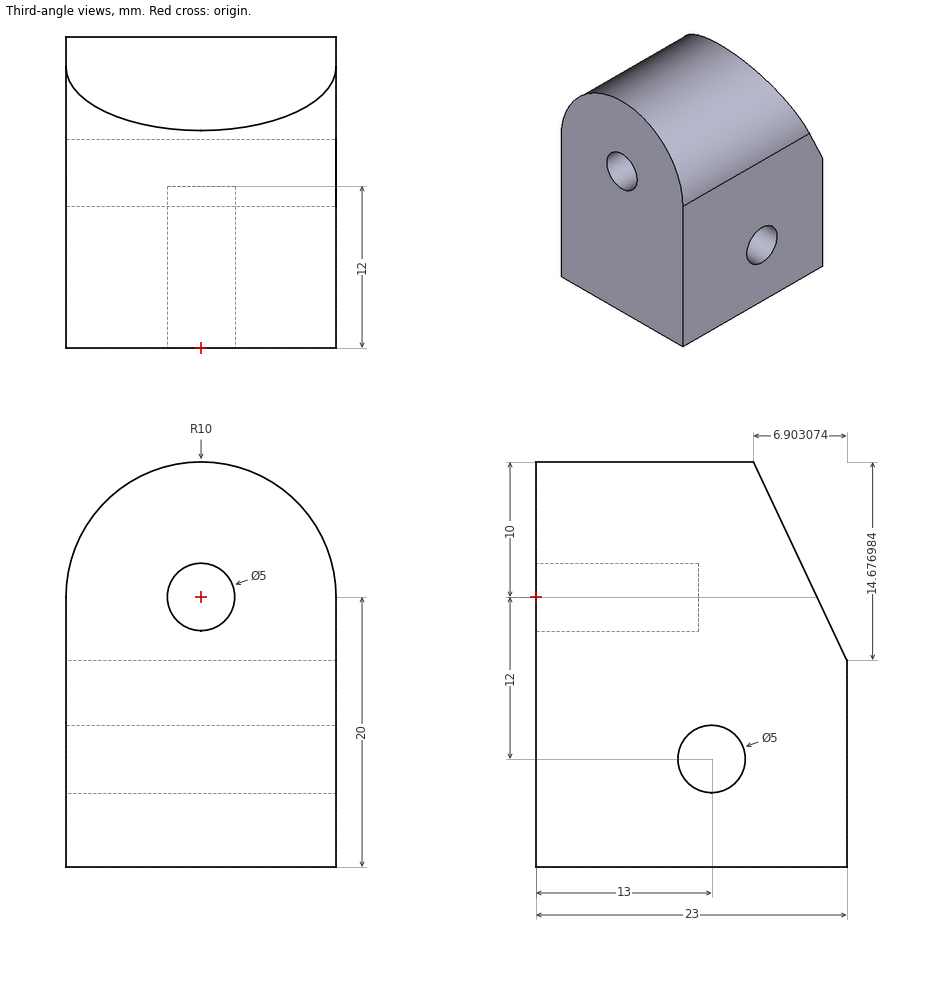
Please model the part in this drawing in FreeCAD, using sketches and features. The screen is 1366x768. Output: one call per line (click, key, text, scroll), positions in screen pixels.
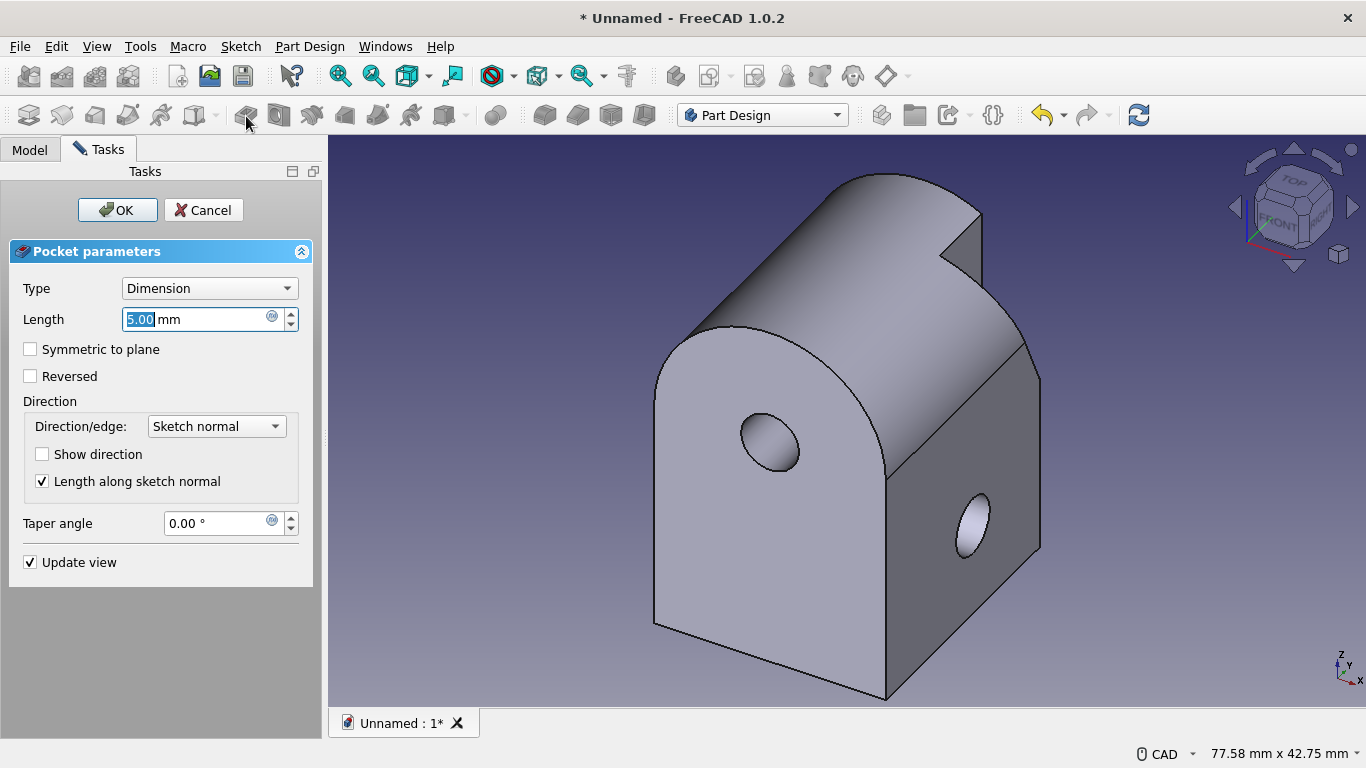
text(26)
key(Tab)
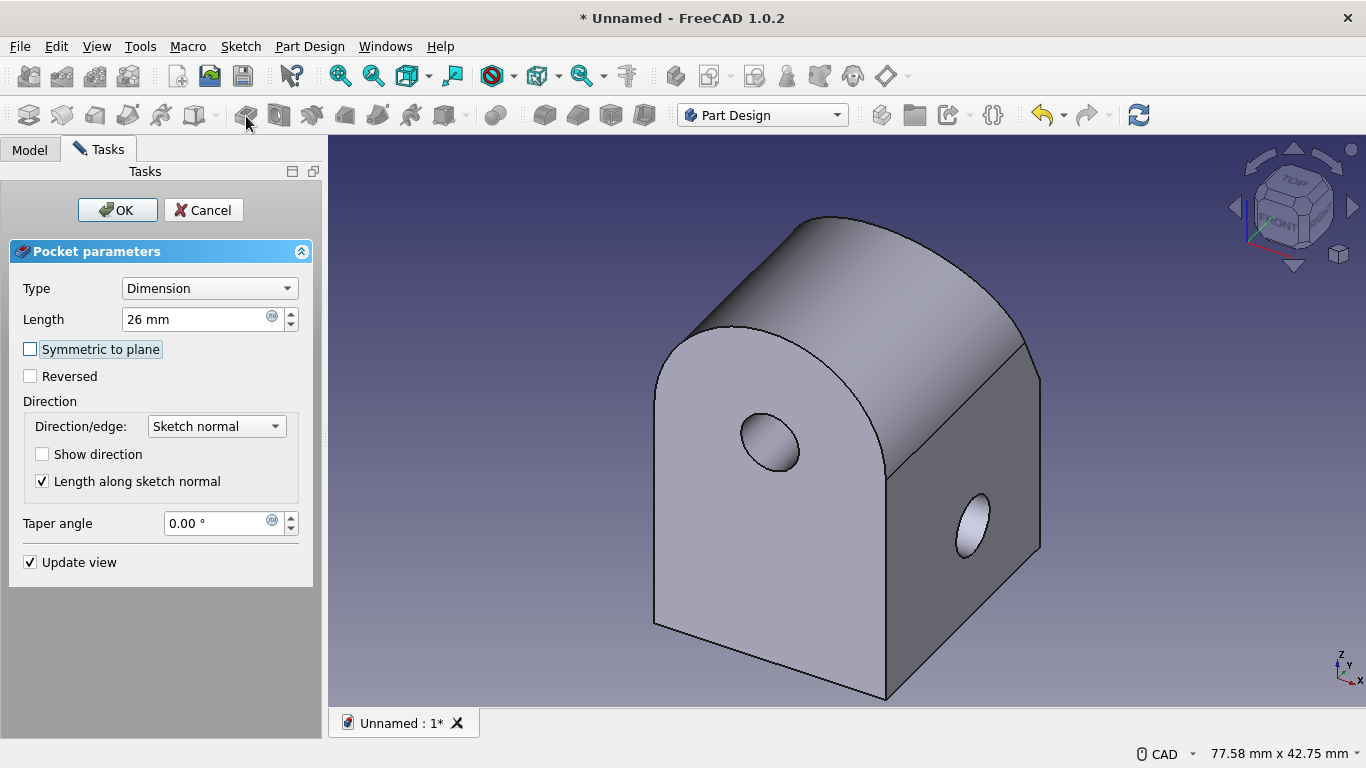
click(118, 210)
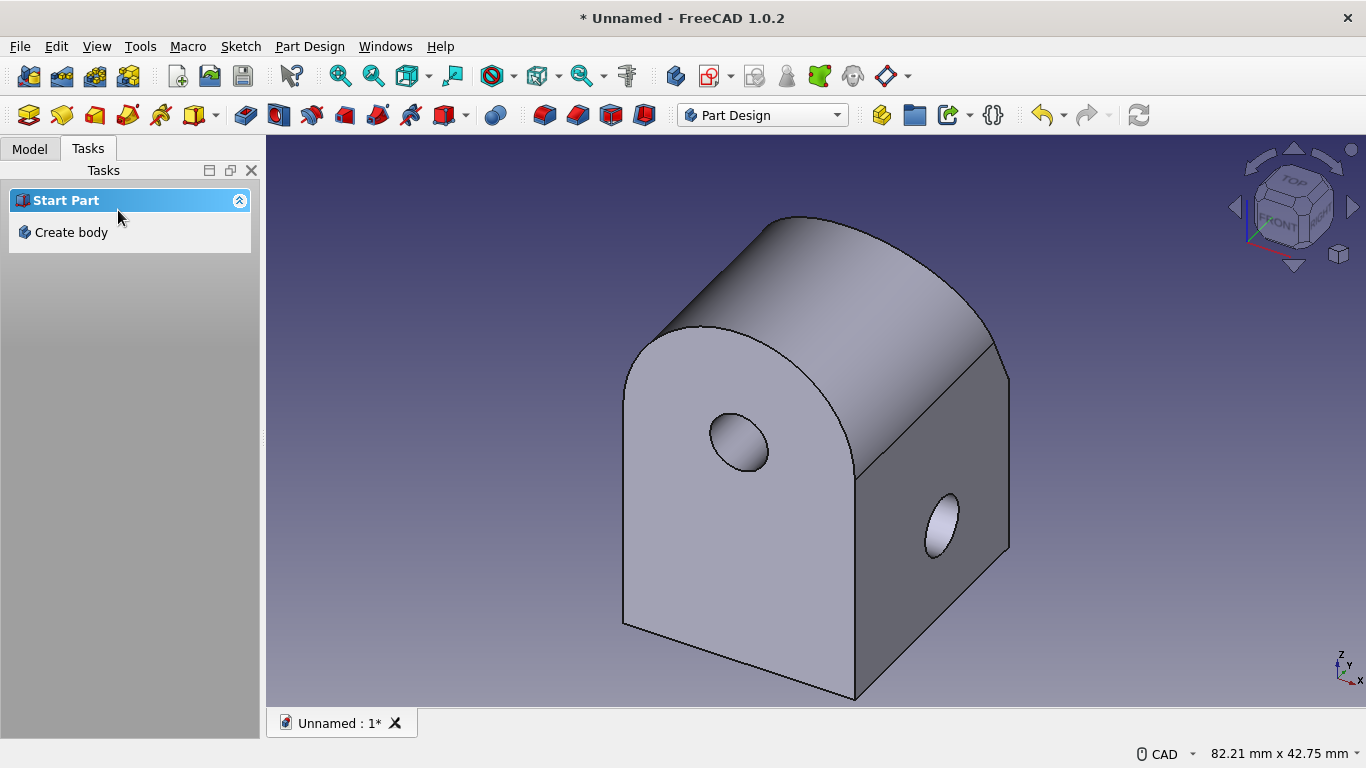
key(0)